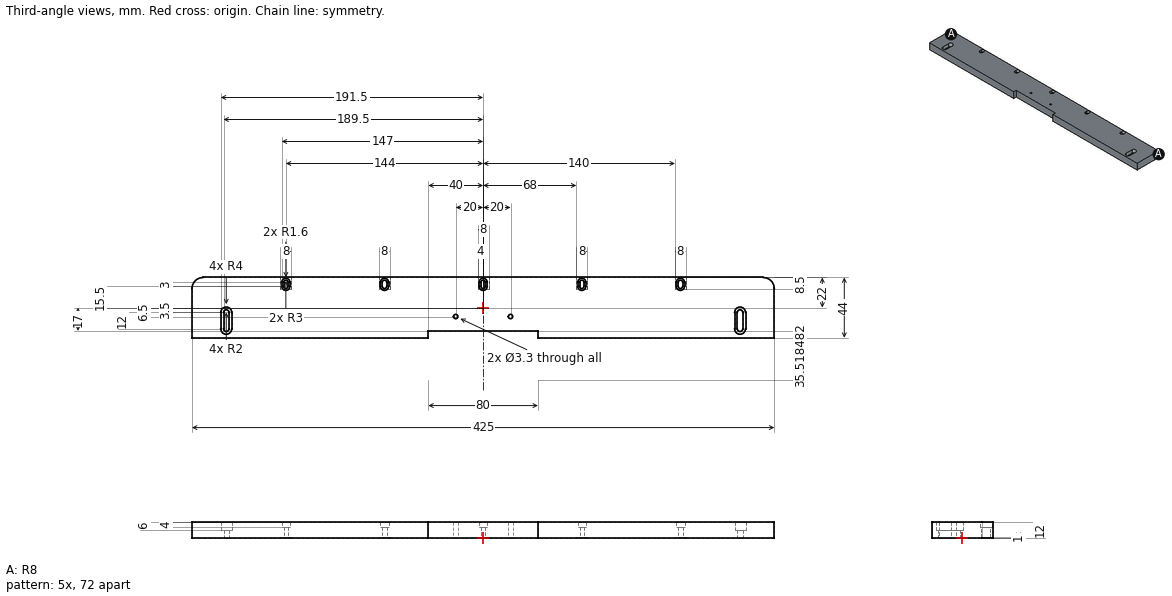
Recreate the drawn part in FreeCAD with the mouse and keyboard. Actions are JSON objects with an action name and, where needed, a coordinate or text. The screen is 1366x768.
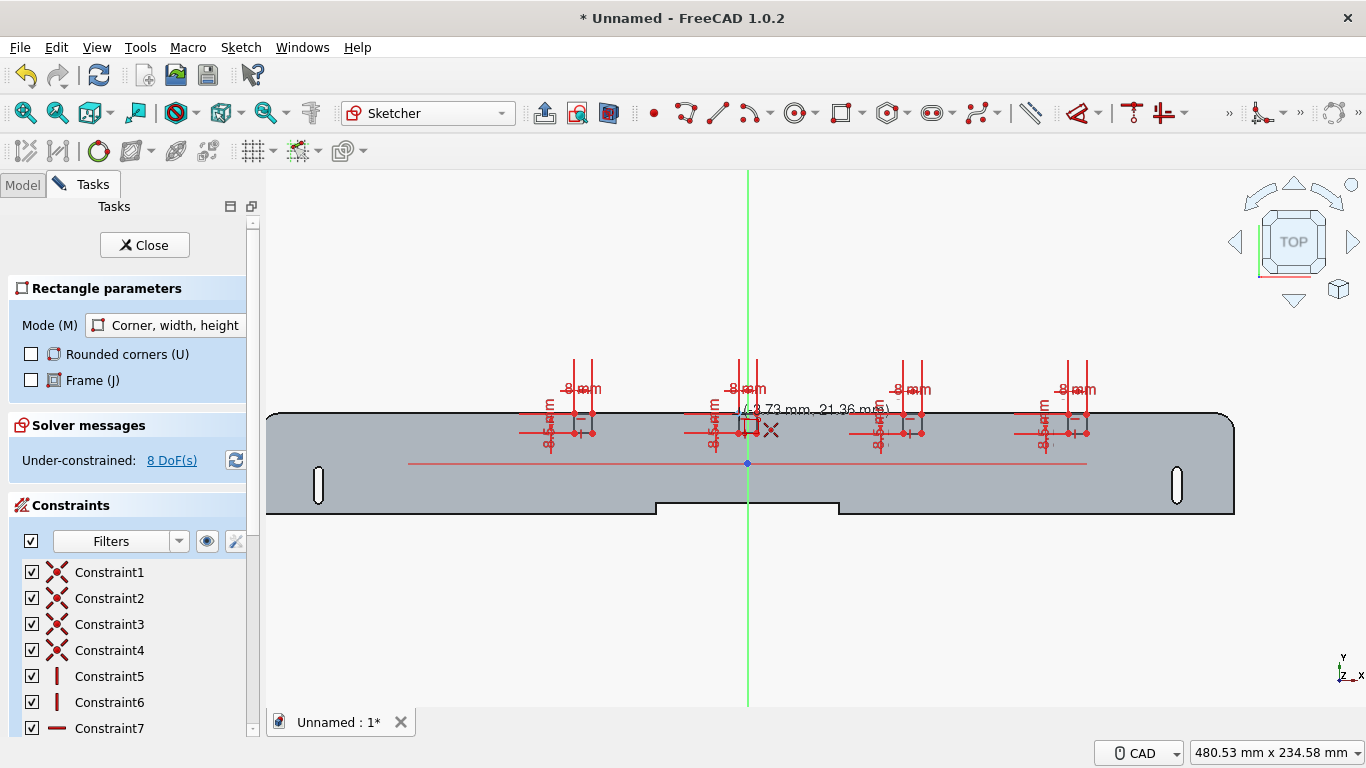
{"action": "left_click", "coordinate": [409, 413]}
{"action": "mouse_move", "coordinate": [427, 433]}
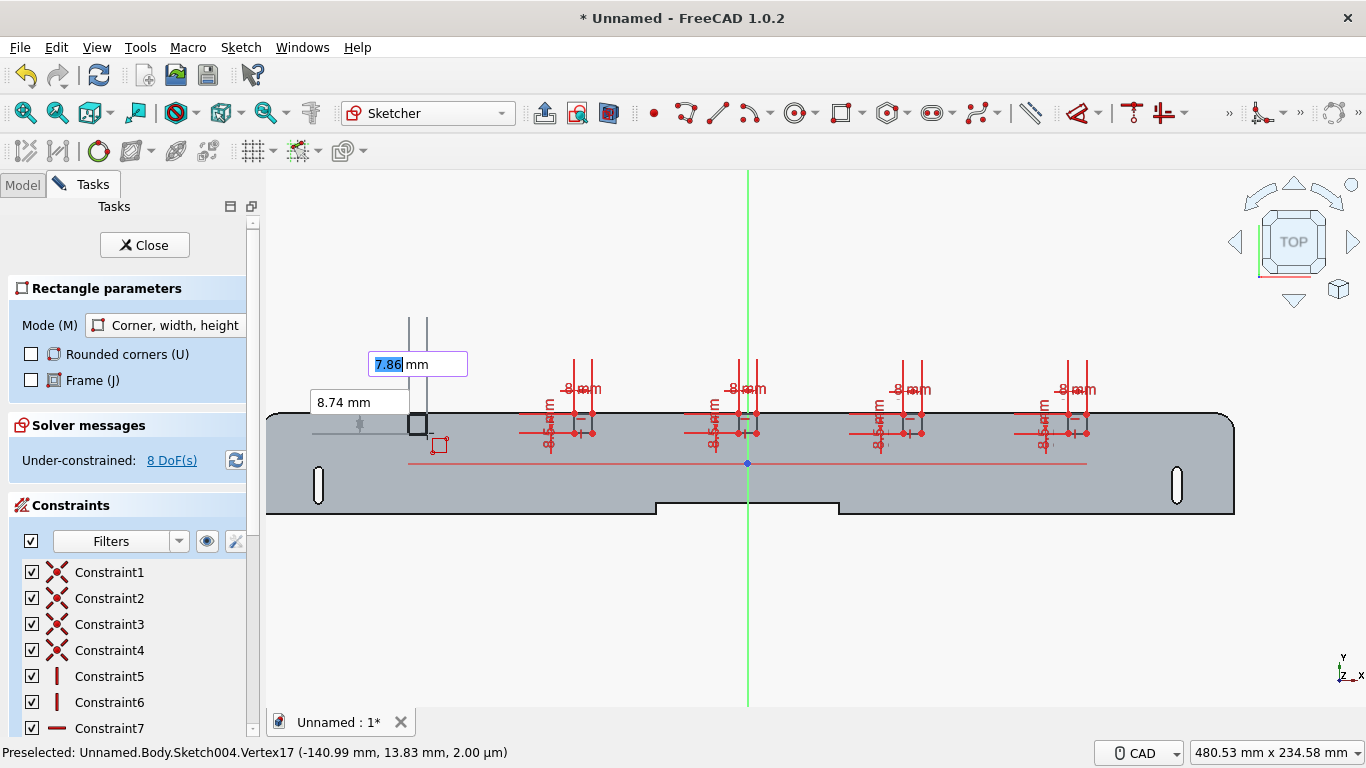
{"action": "type", "text": "8"}
{"action": "key", "text": "Tab"}
{"action": "type", "text": "8.5"}
{"action": "key", "text": "Return"}
{"action": "key", "text": "Escape"}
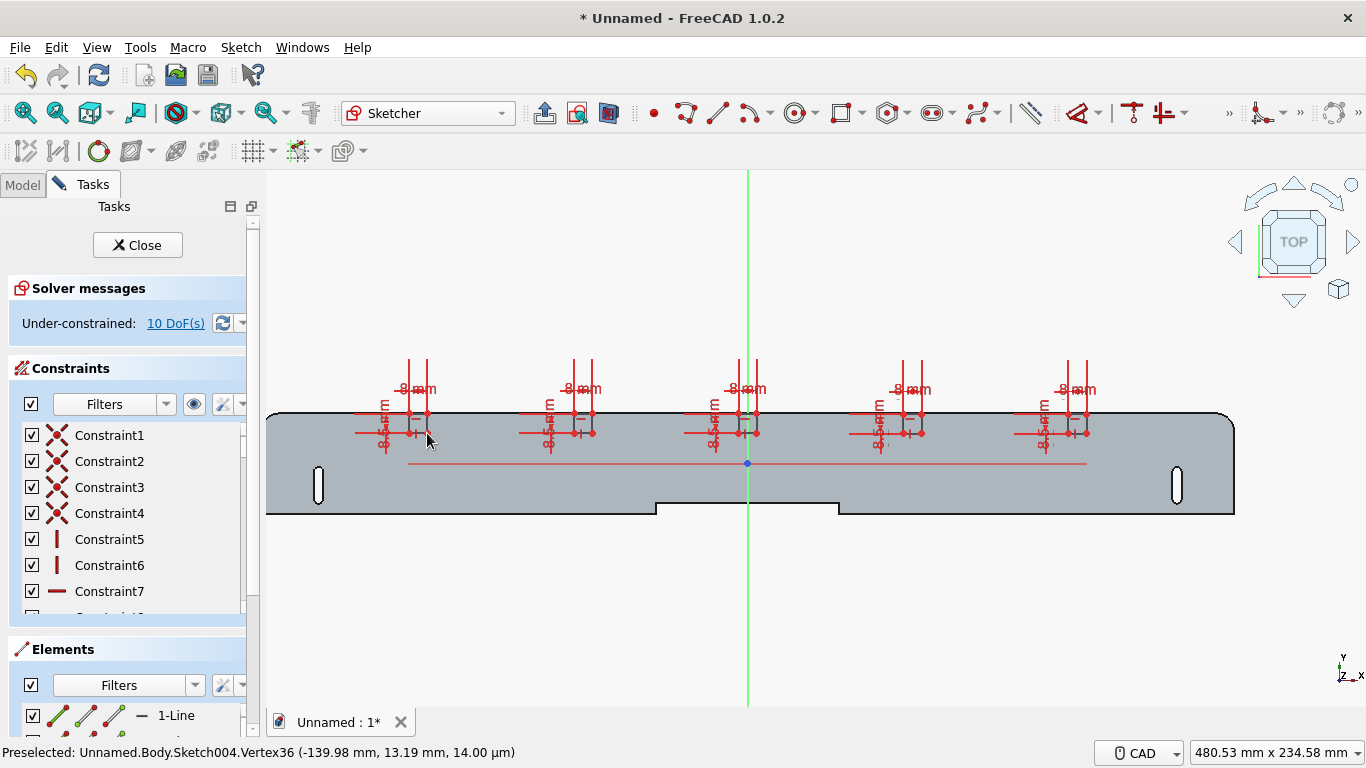
{"action": "left_click", "coordinate": [922, 414]}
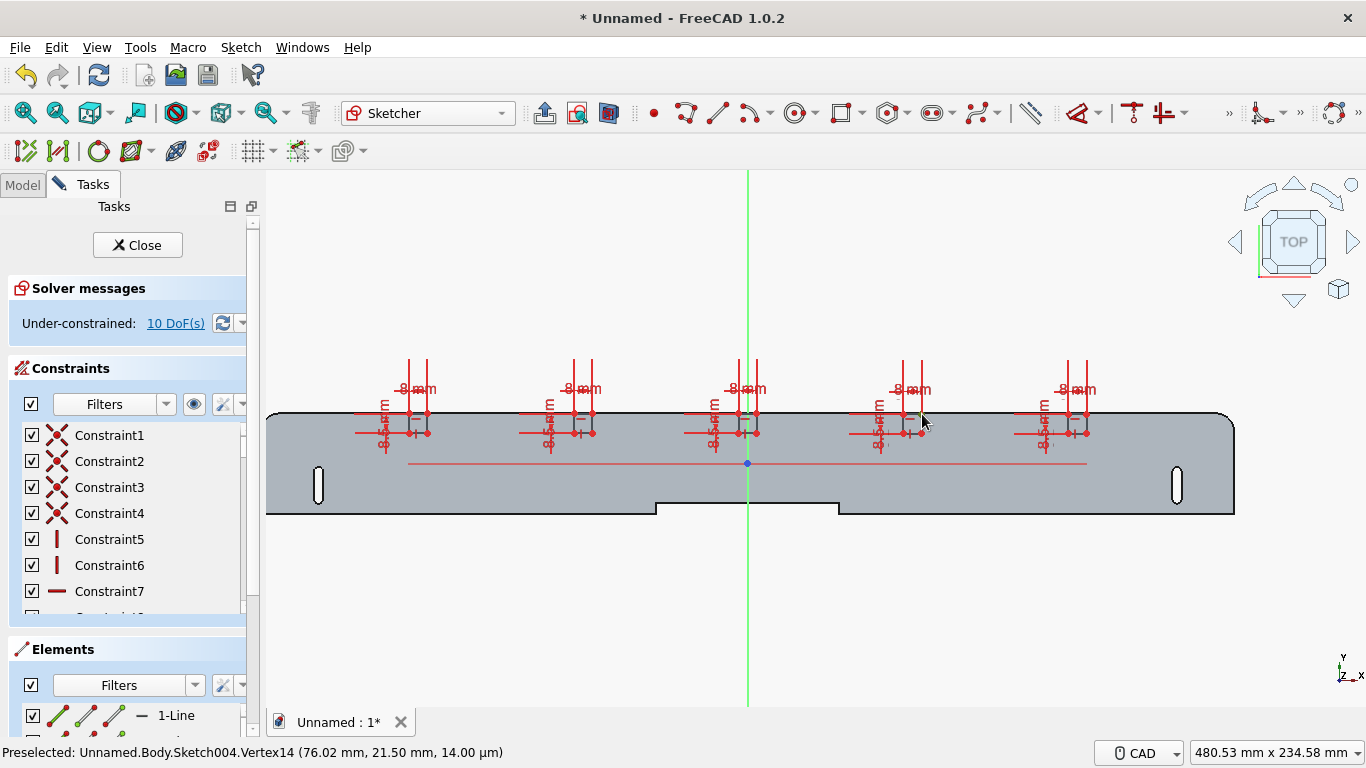
{"action": "left_click", "coordinate": [574, 414]}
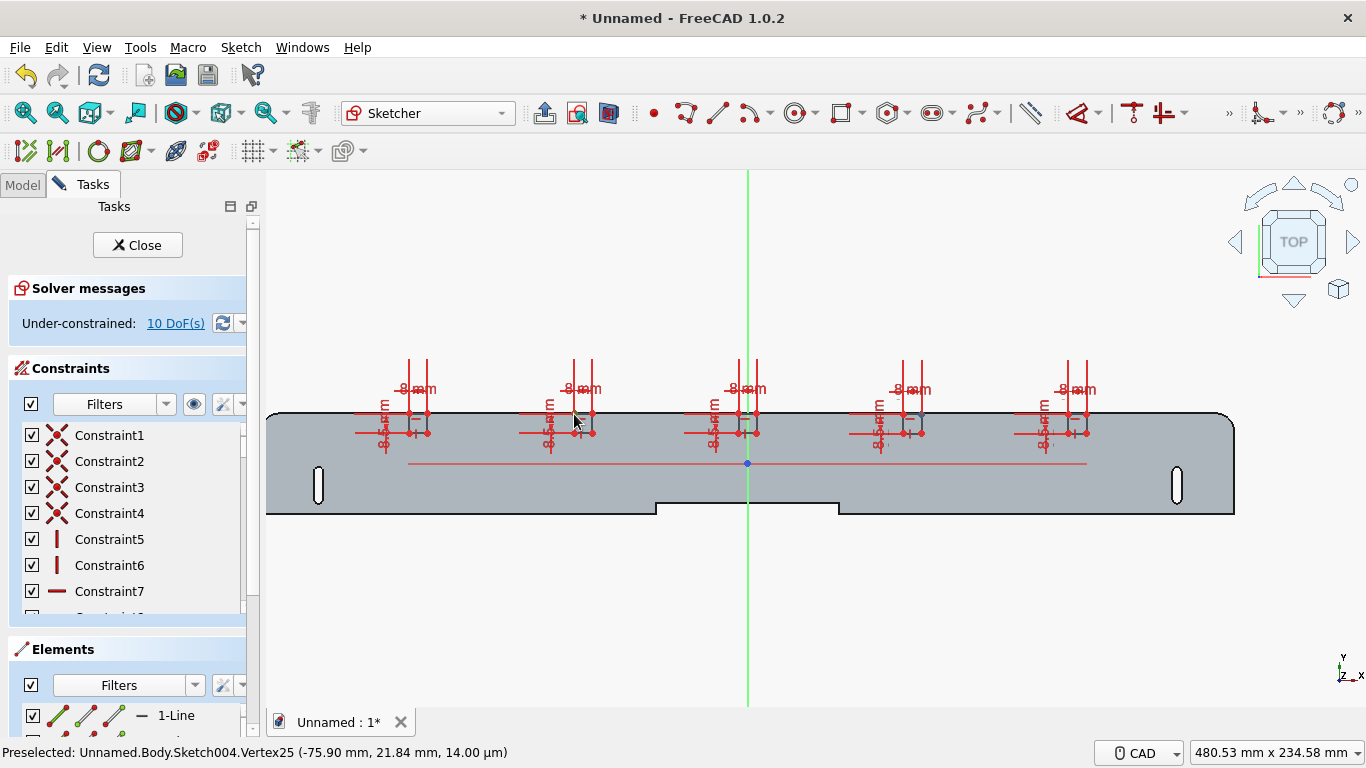
{"action": "left_click", "coordinate": [748, 645]}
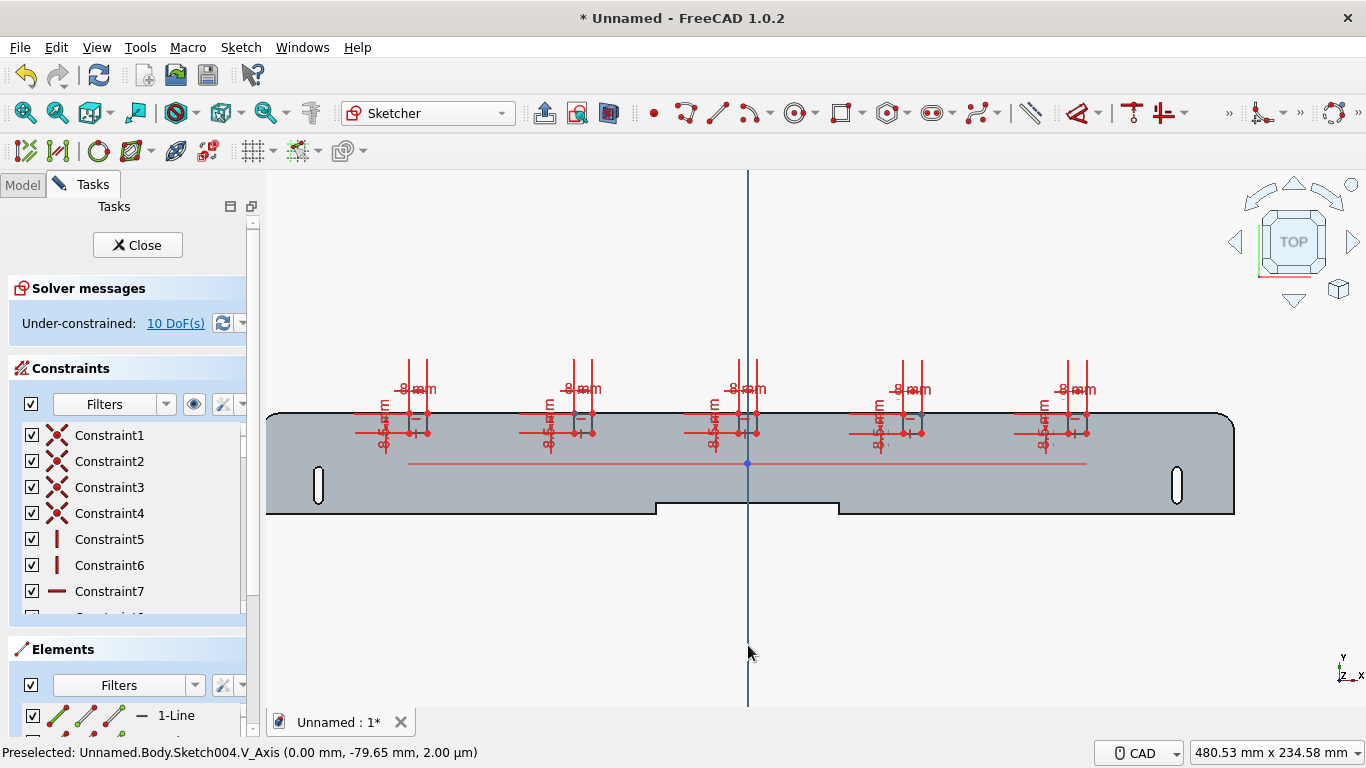
{"action": "key", "text": "s"}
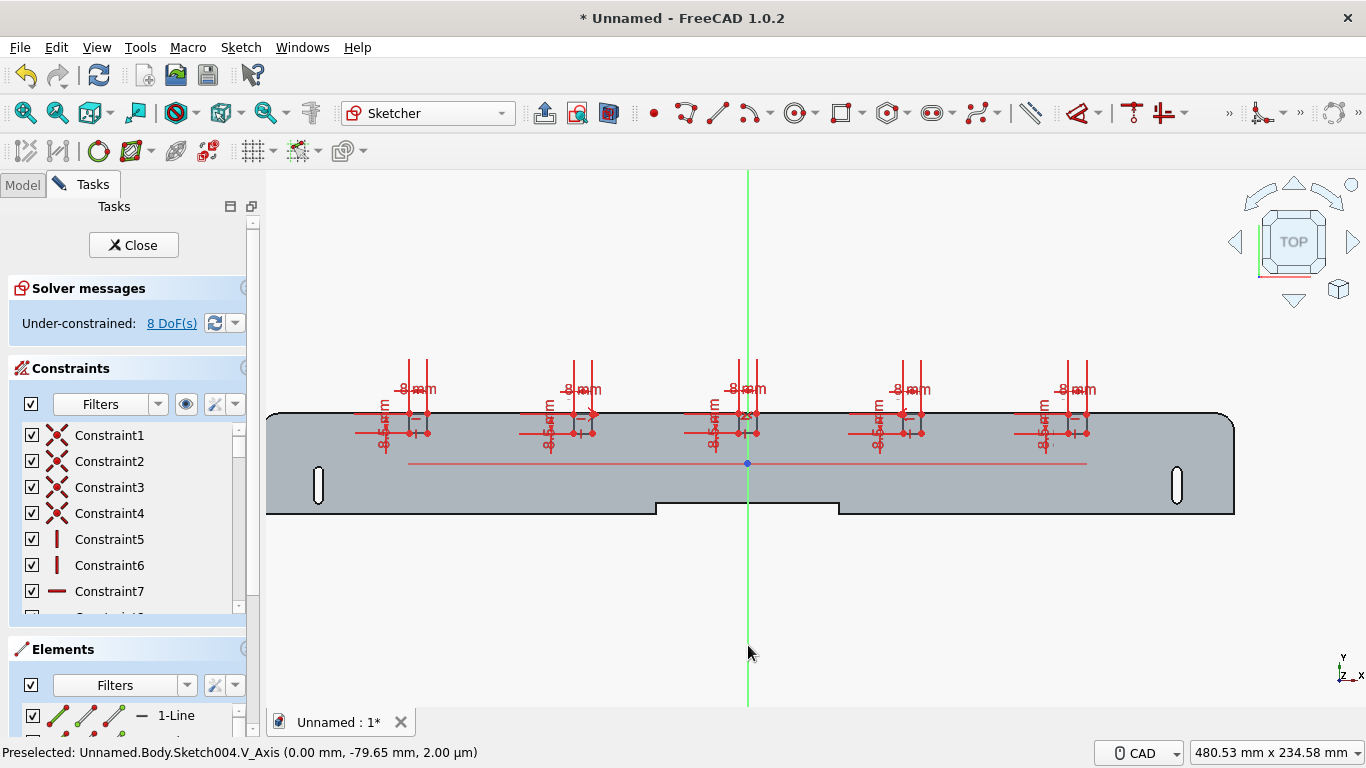
{"action": "left_click", "coordinate": [1087, 414]}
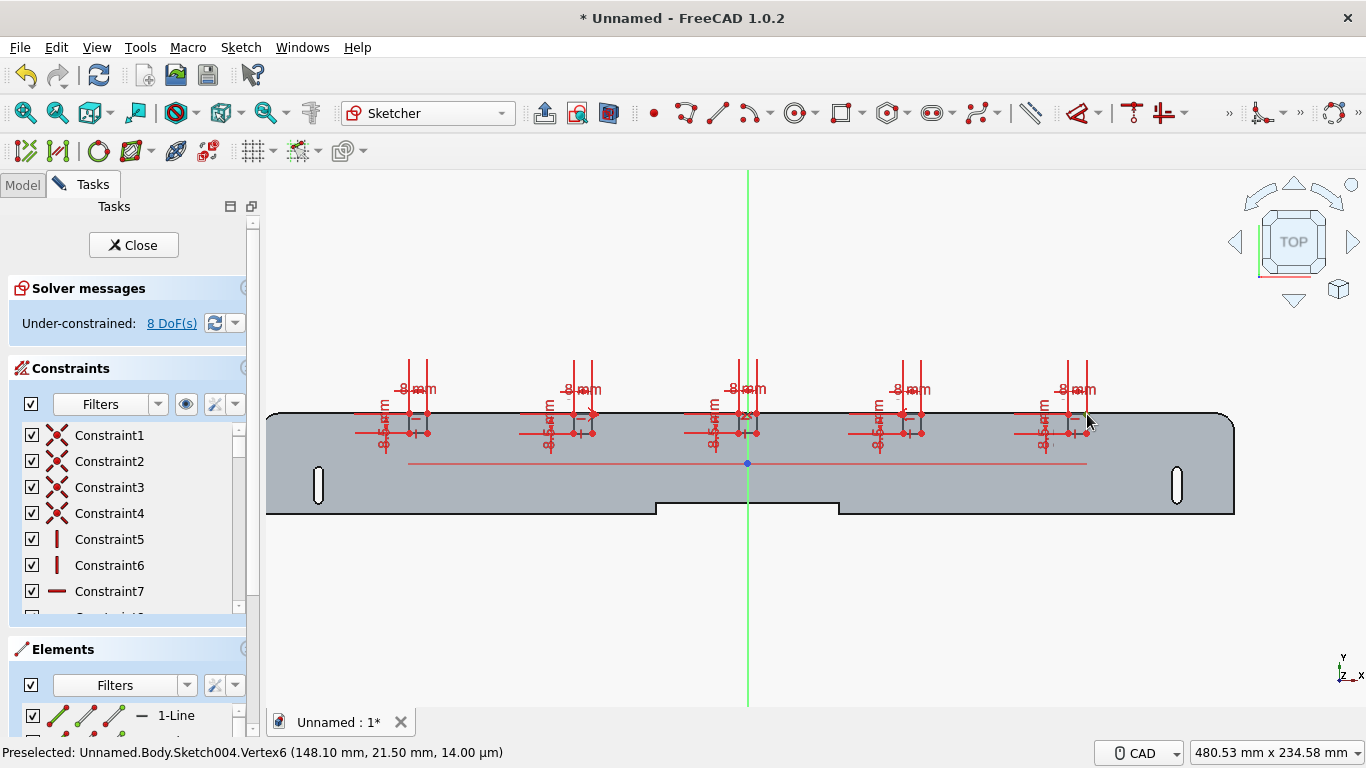
{"action": "left_click", "coordinate": [409, 414]}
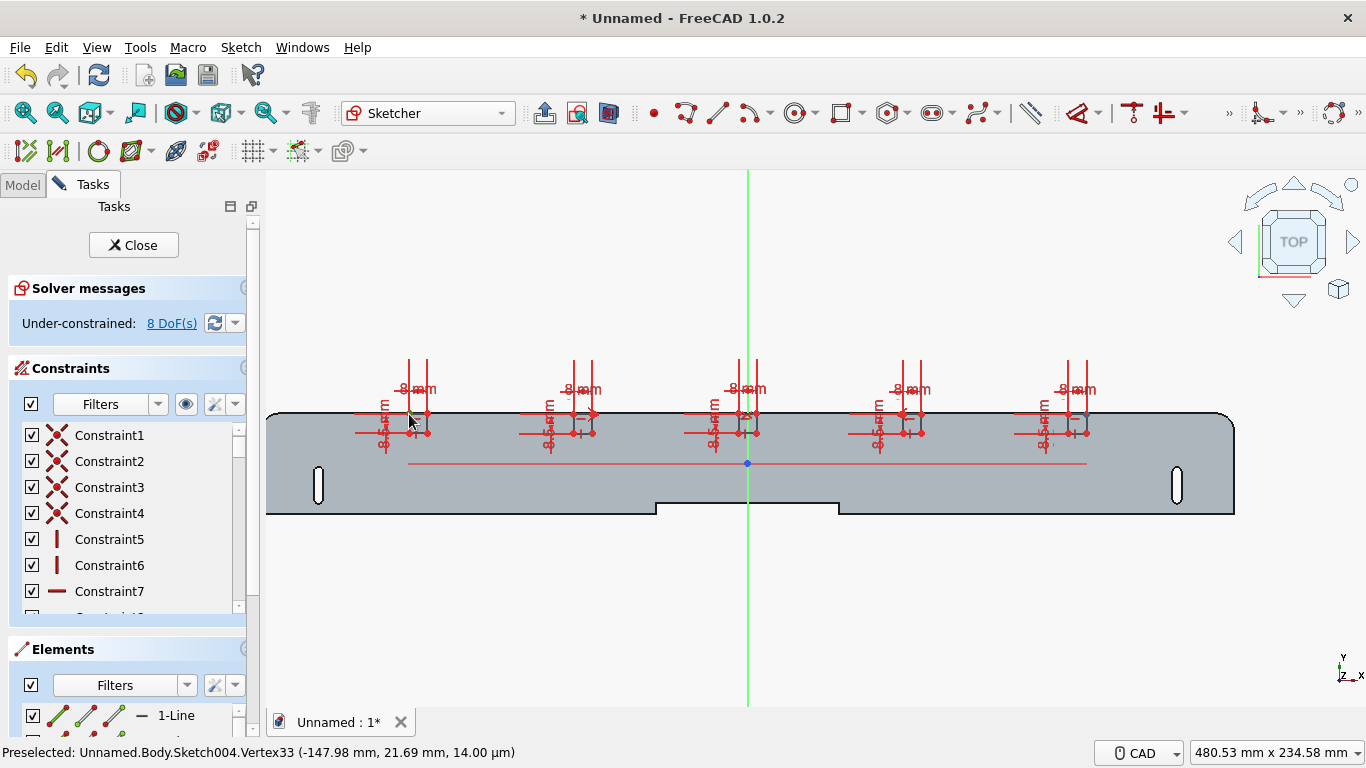
{"action": "left_click", "coordinate": [748, 645]}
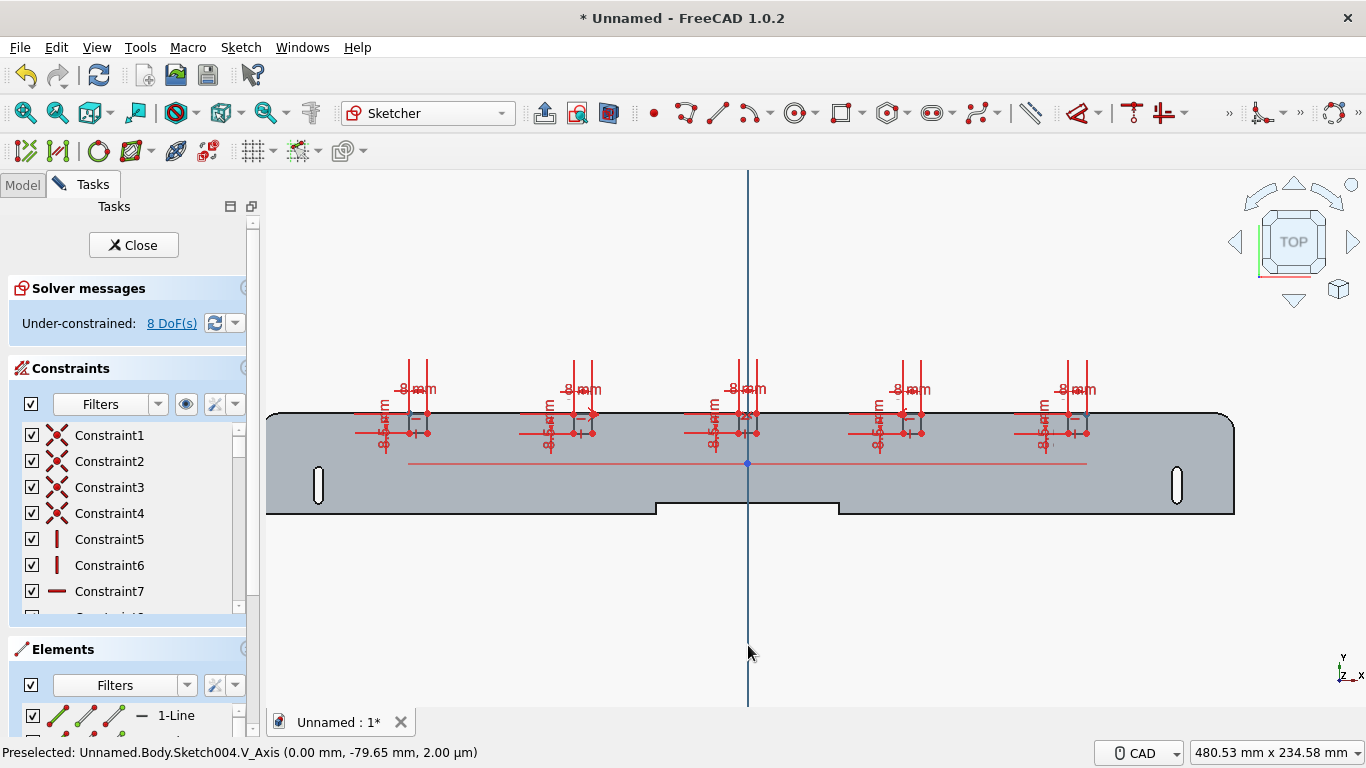
{"action": "key", "text": "s"}